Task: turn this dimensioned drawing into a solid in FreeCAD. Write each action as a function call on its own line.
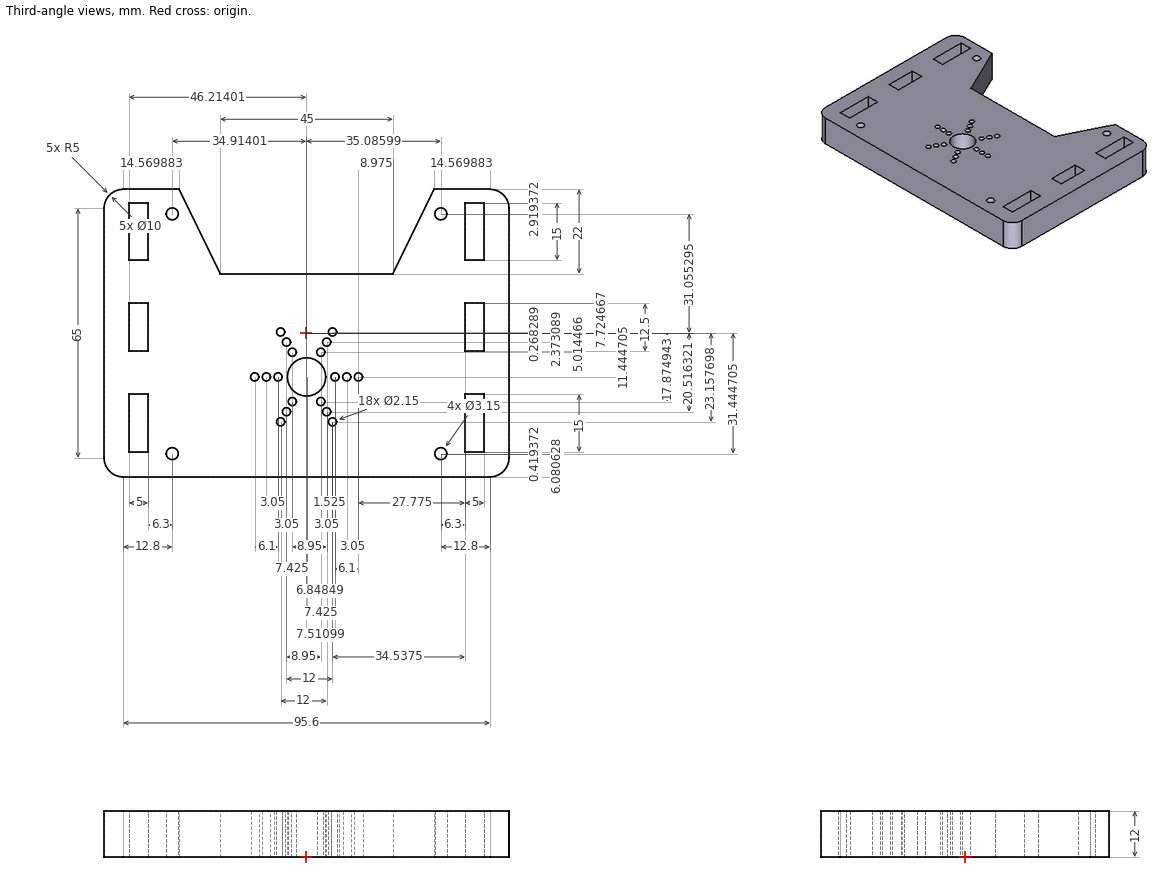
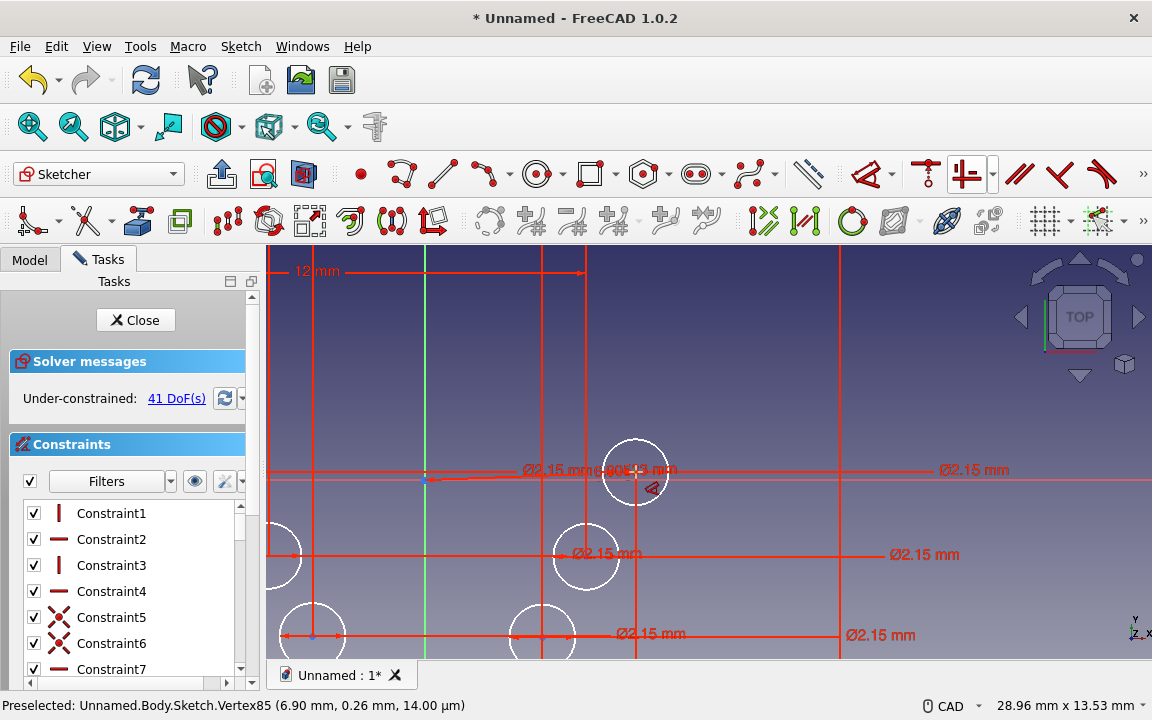
click(586, 557)
click(622, 591)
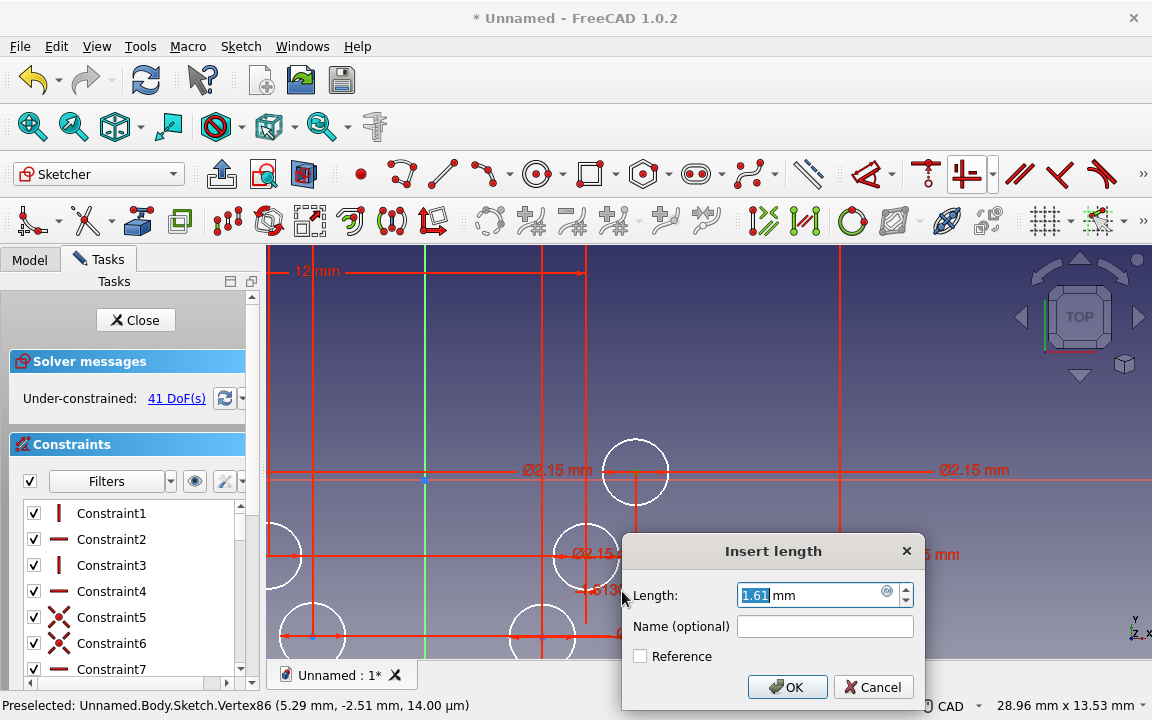
text(1.525)
key(Return)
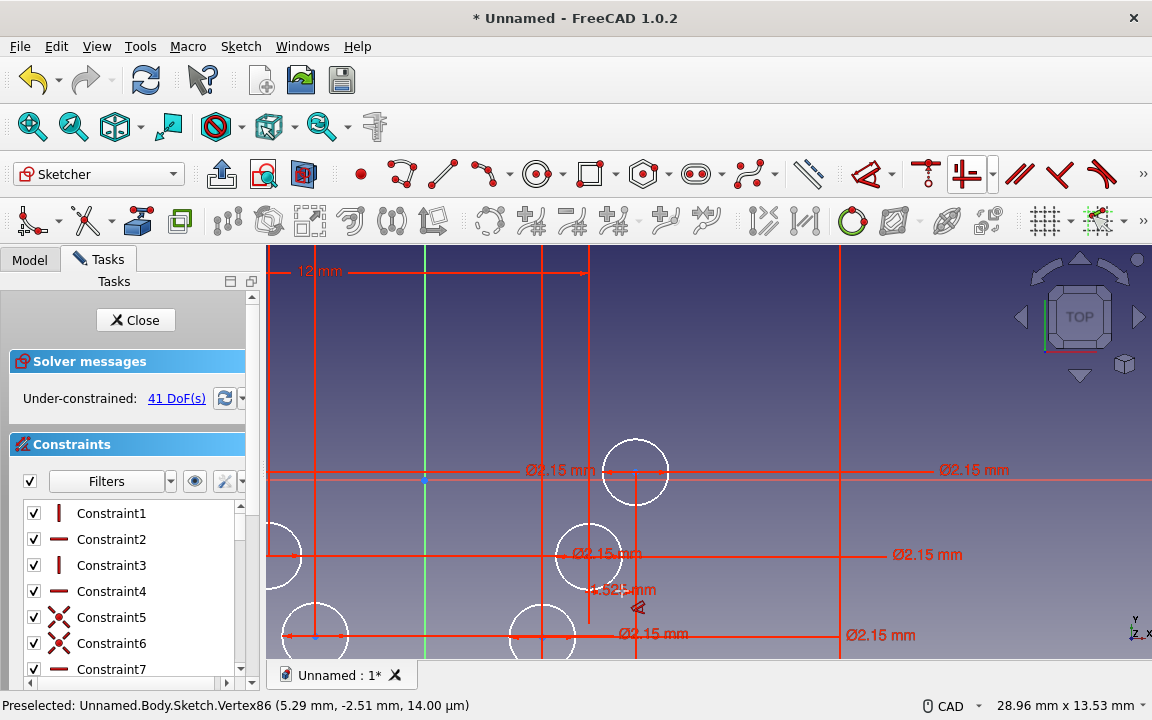
scroll(667, 448, down, 11)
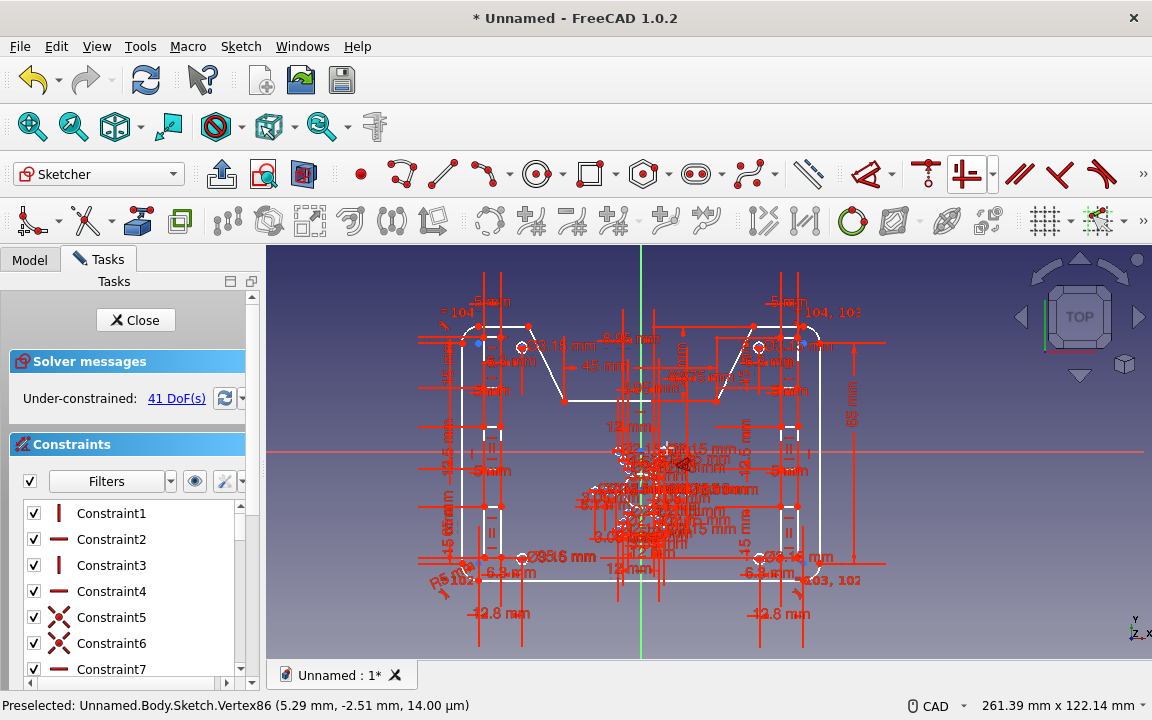
scroll(666, 491, up, 3)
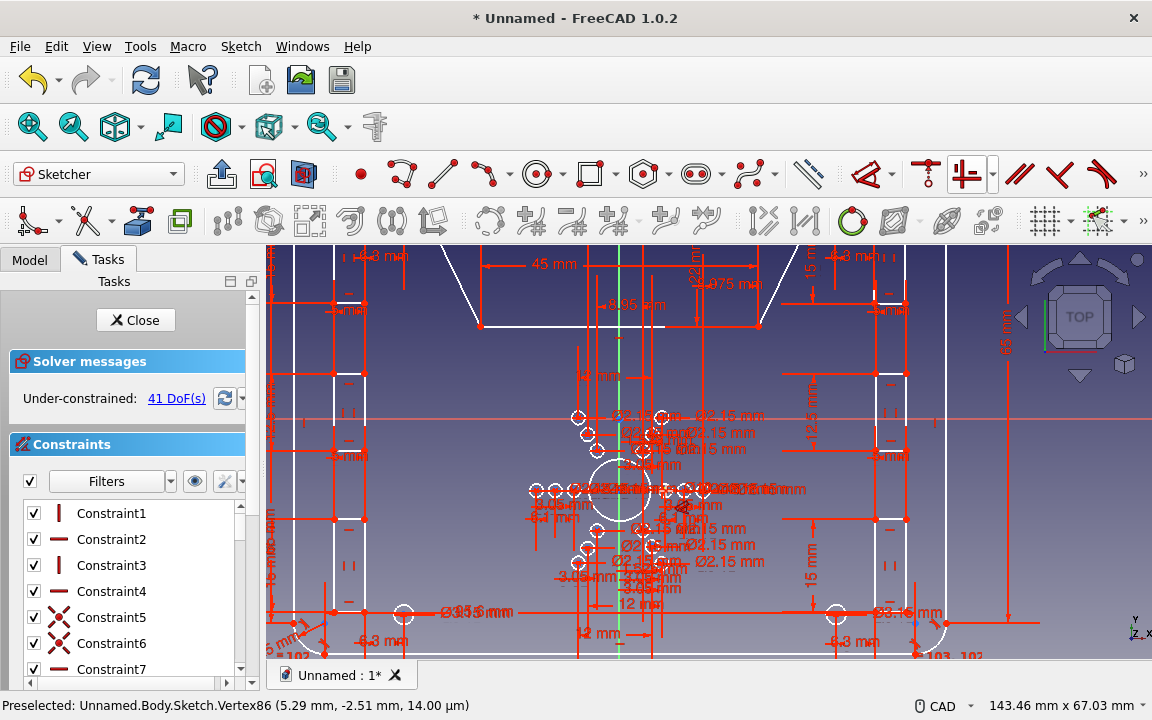
click(665, 491)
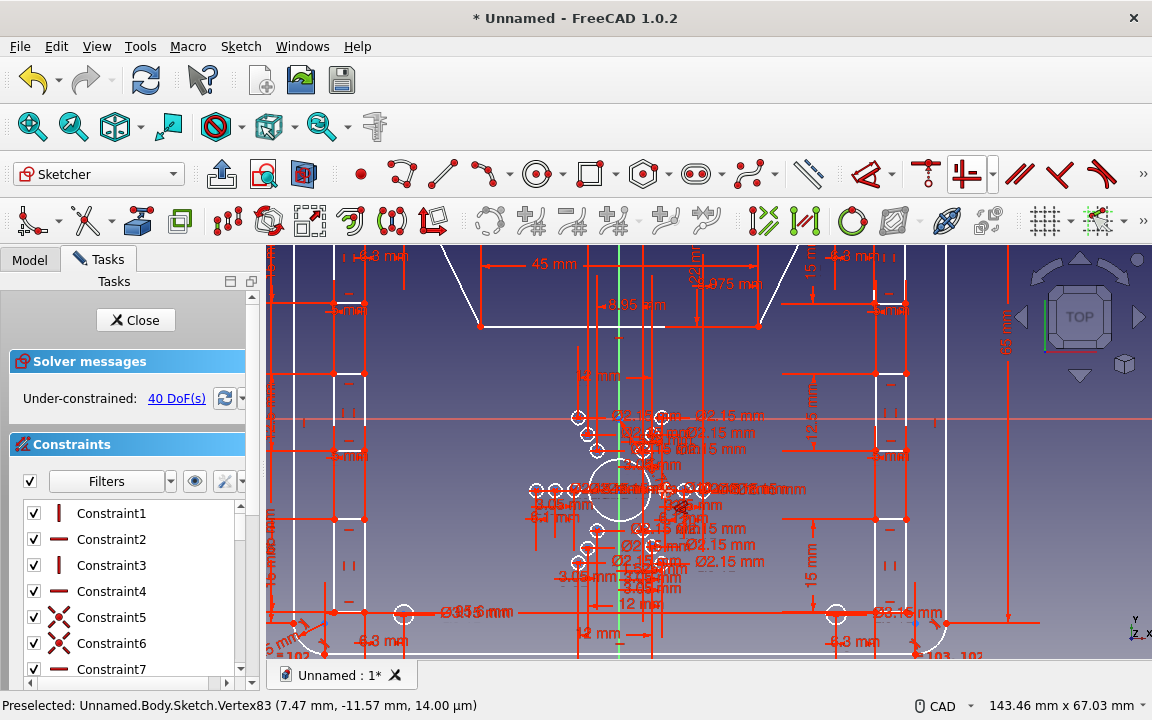
click(620, 490)
click(659, 456)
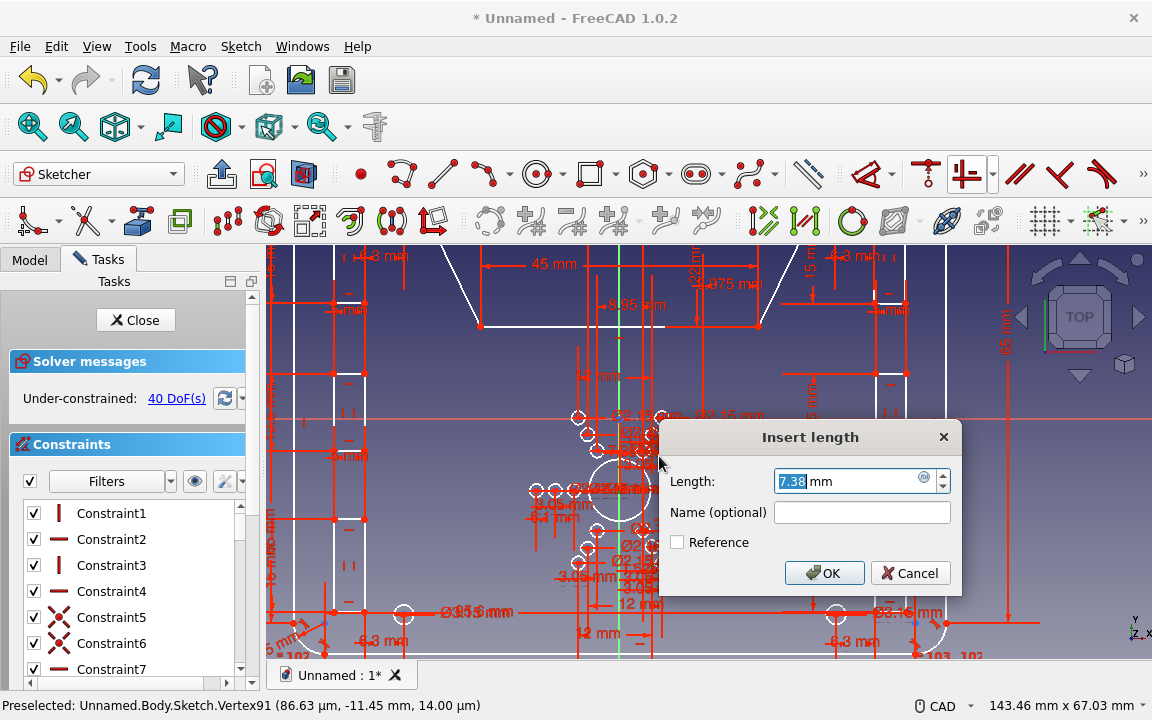
text(7.425)
key(Return)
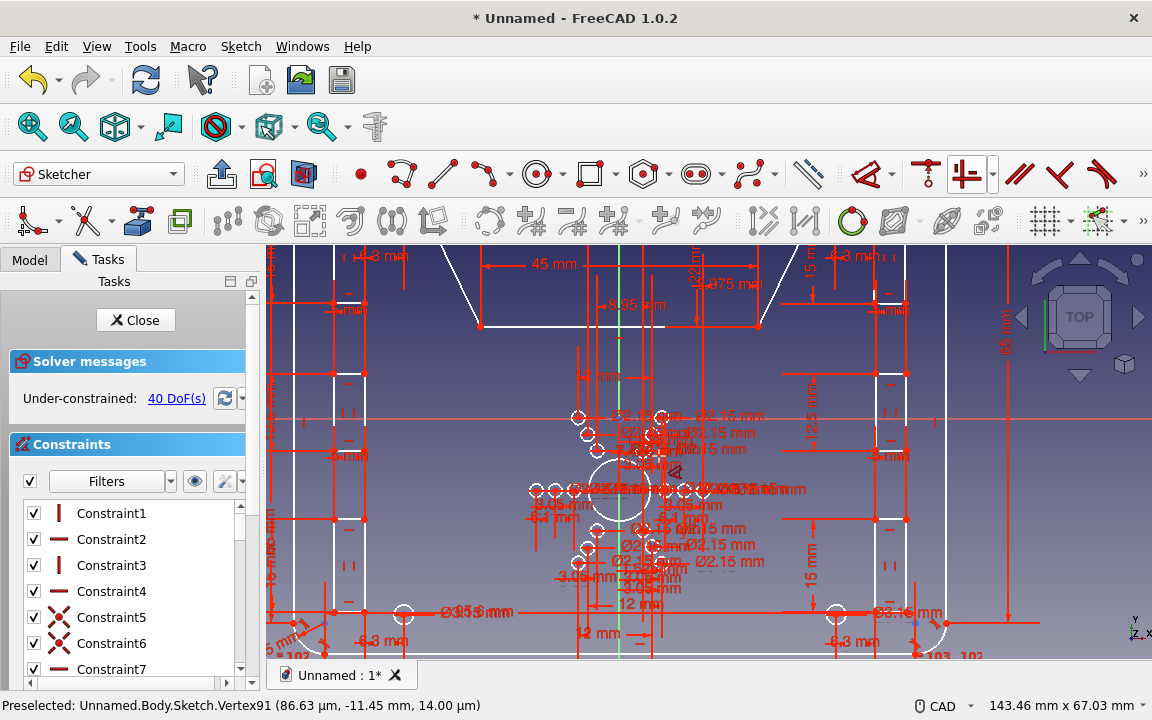
click(619, 490)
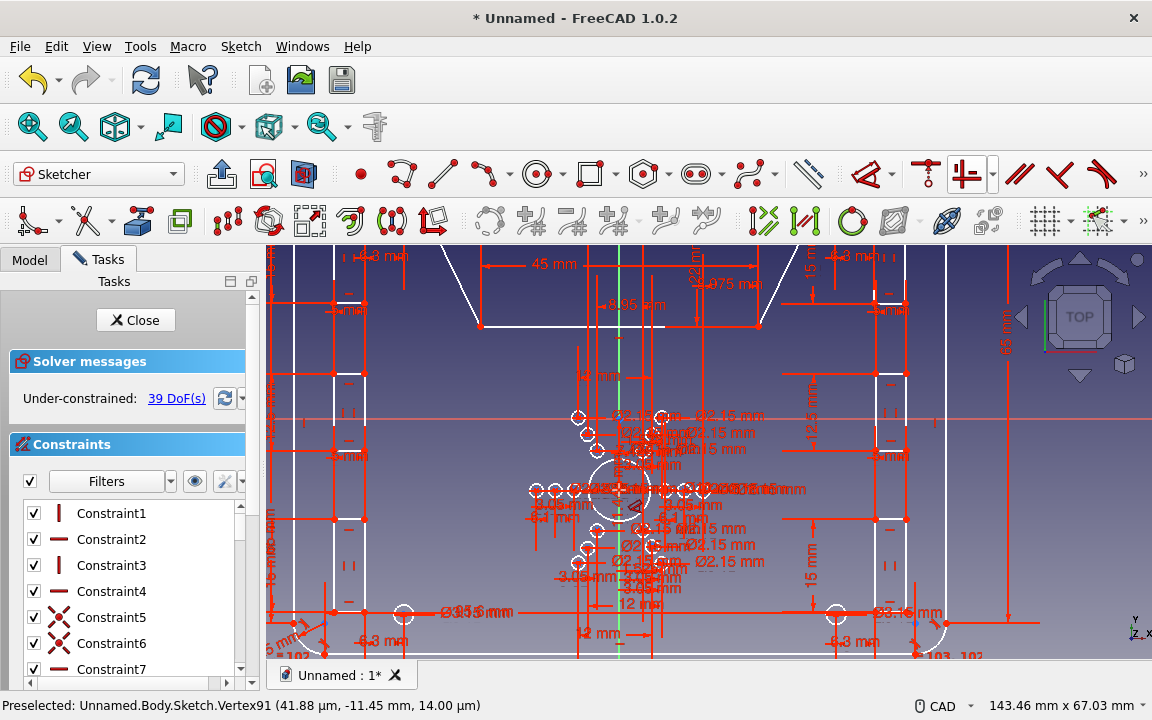
click(574, 491)
click(581, 456)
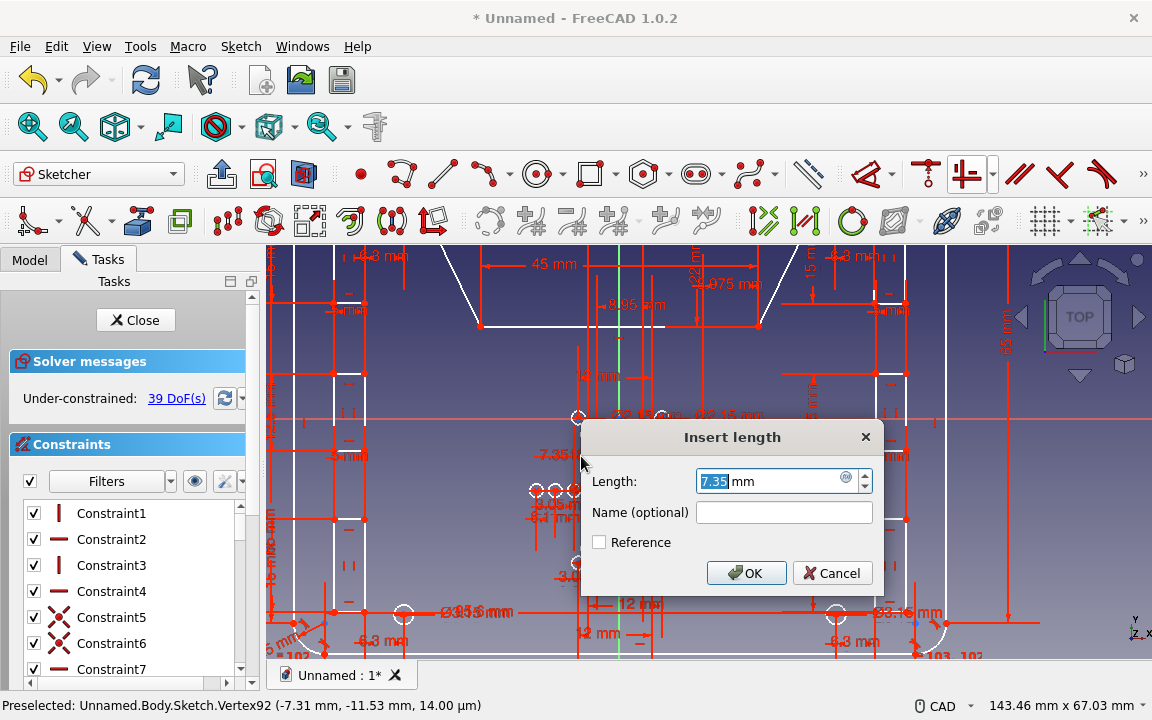
text(7.425)
key(Return)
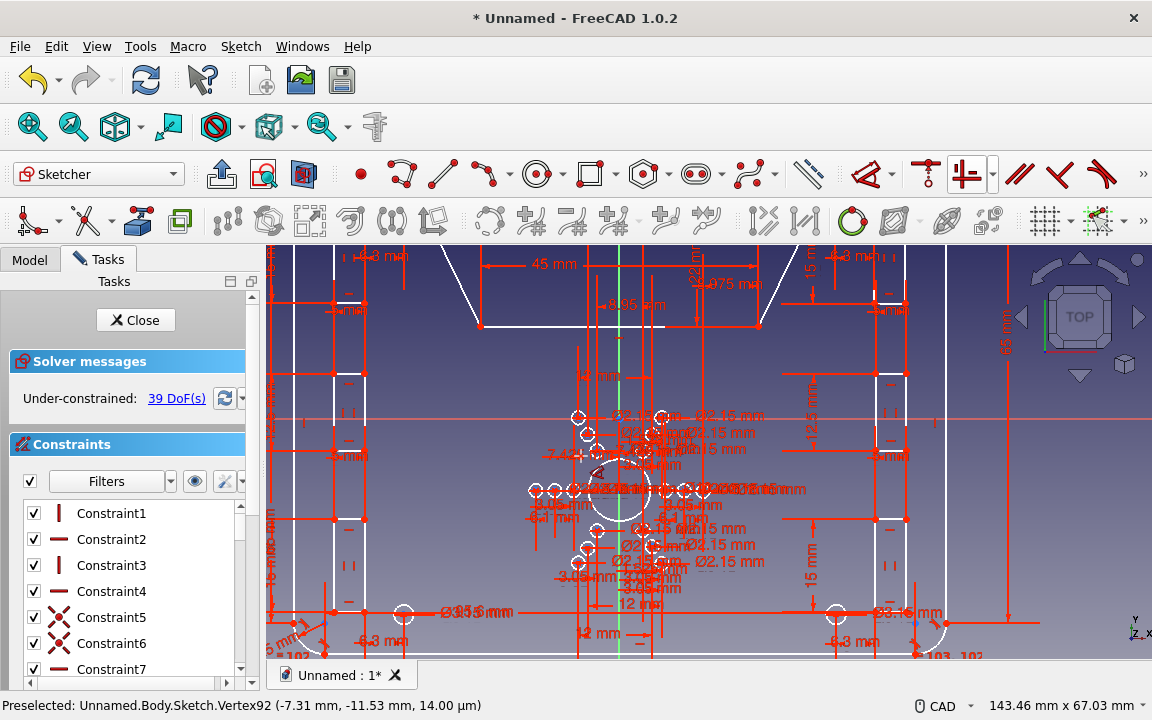
click(662, 564)
click(641, 385)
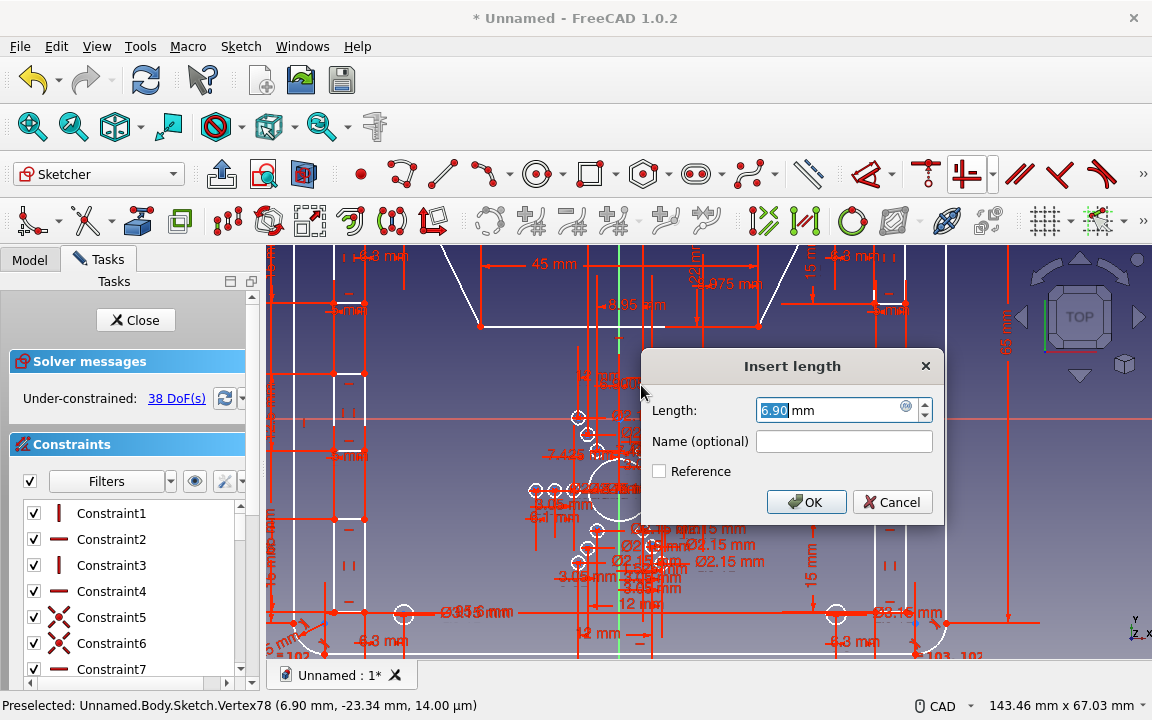
text(6.84849)
key(Return)